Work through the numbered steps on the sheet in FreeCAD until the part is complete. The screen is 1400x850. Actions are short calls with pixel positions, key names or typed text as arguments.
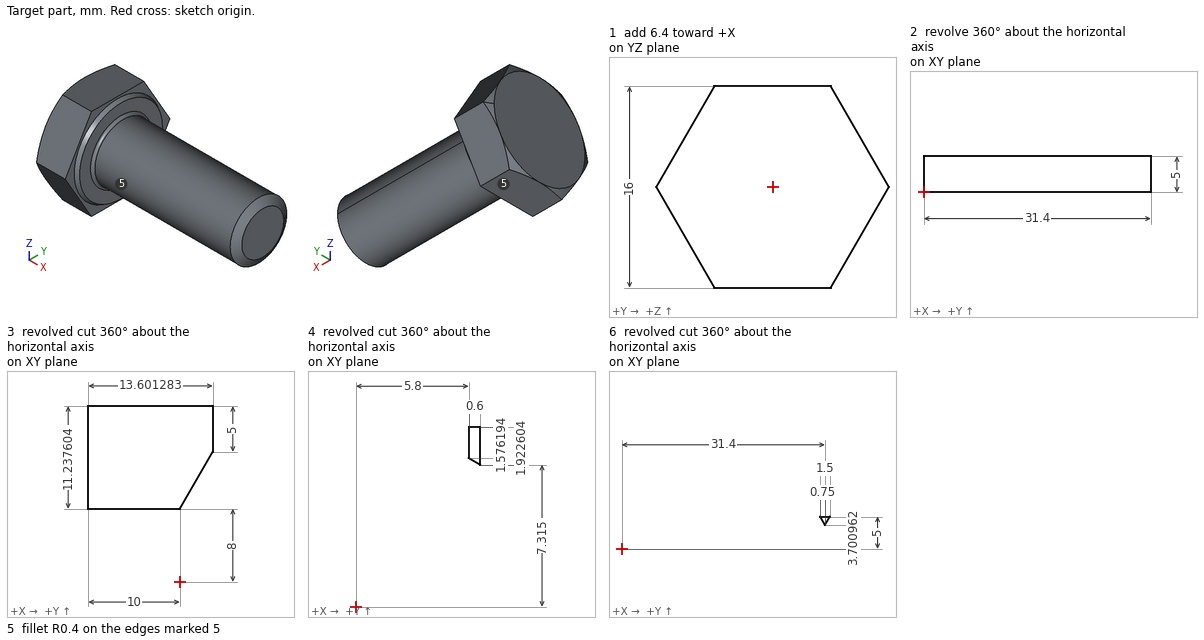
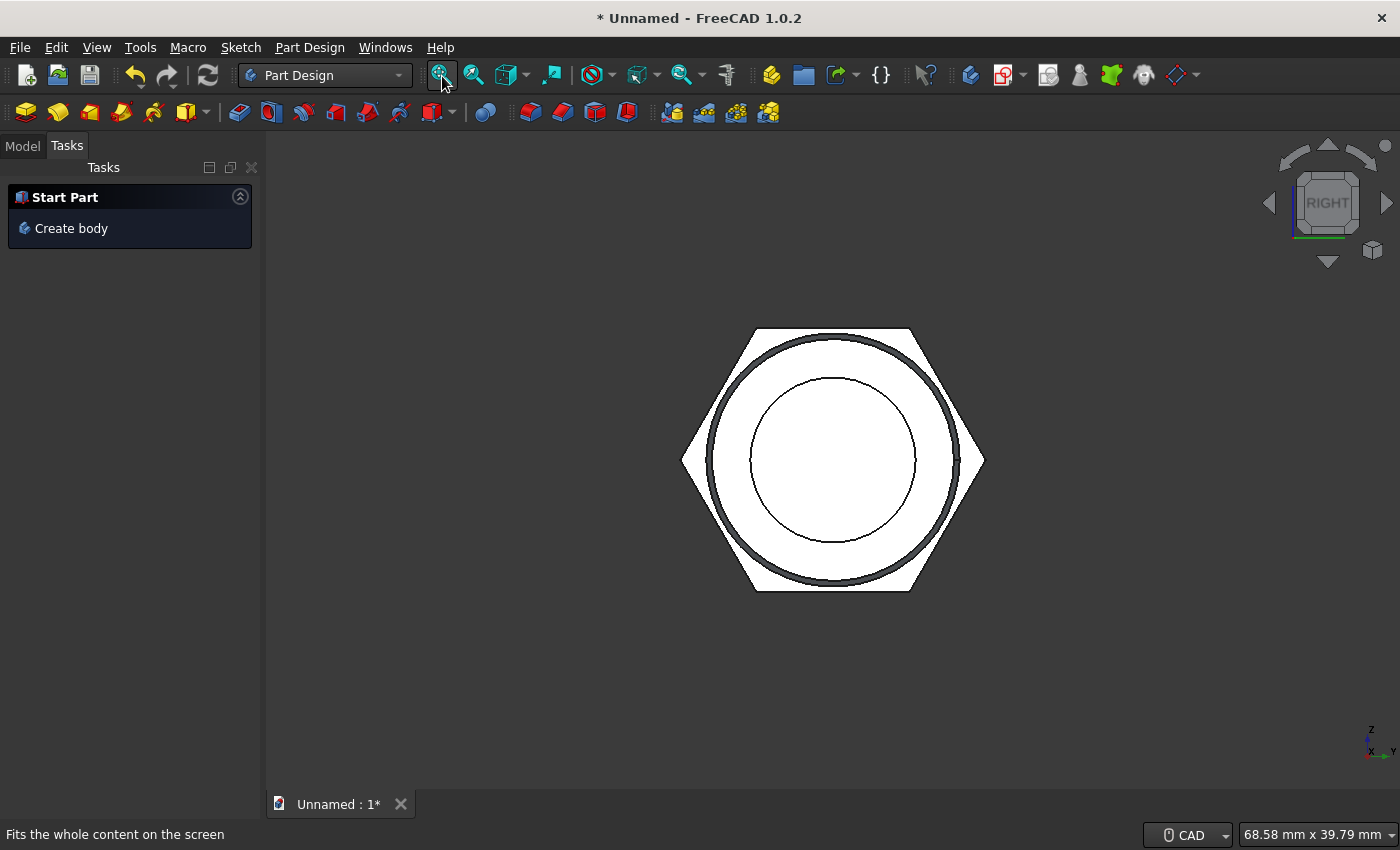
key(5)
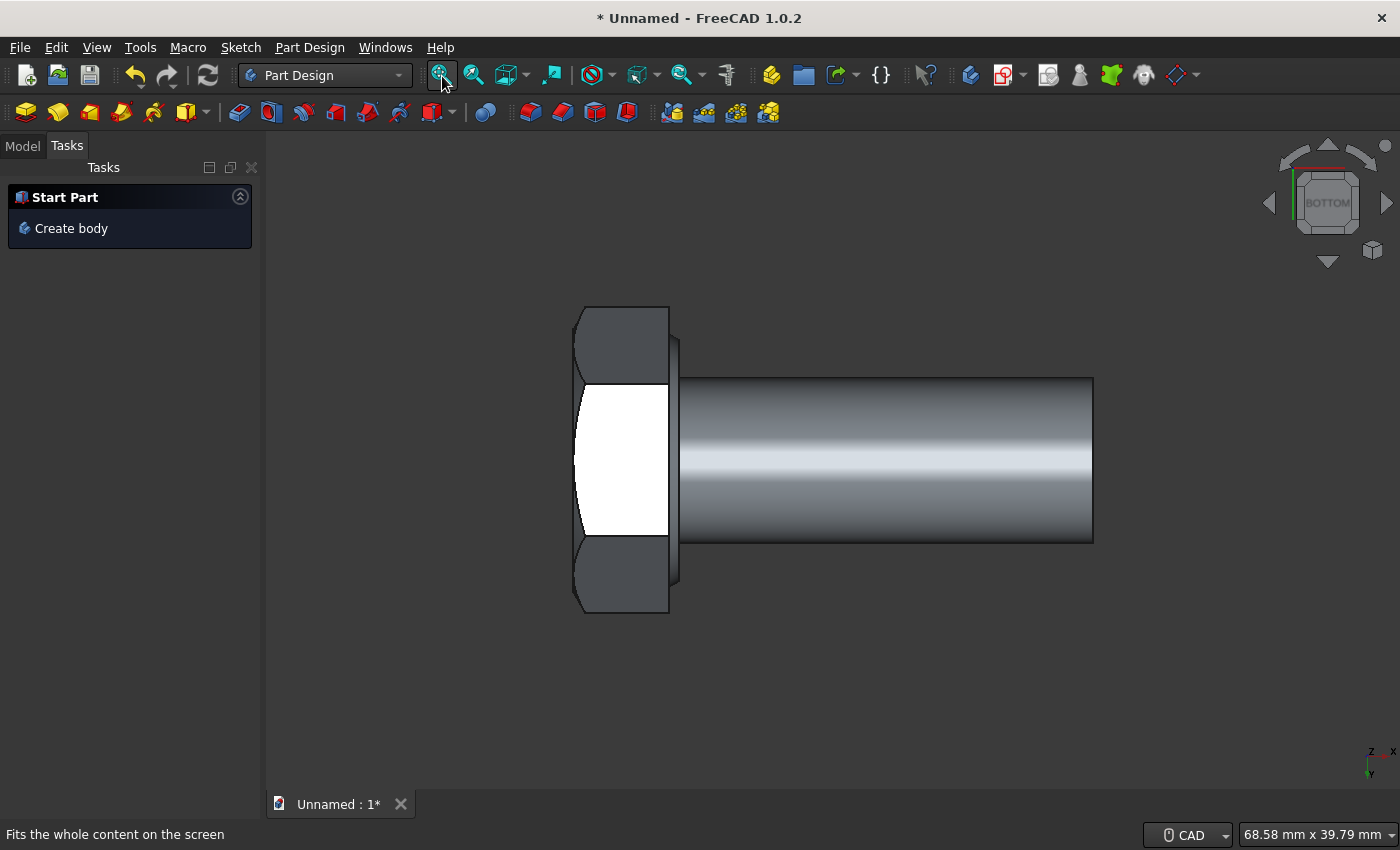
key(4)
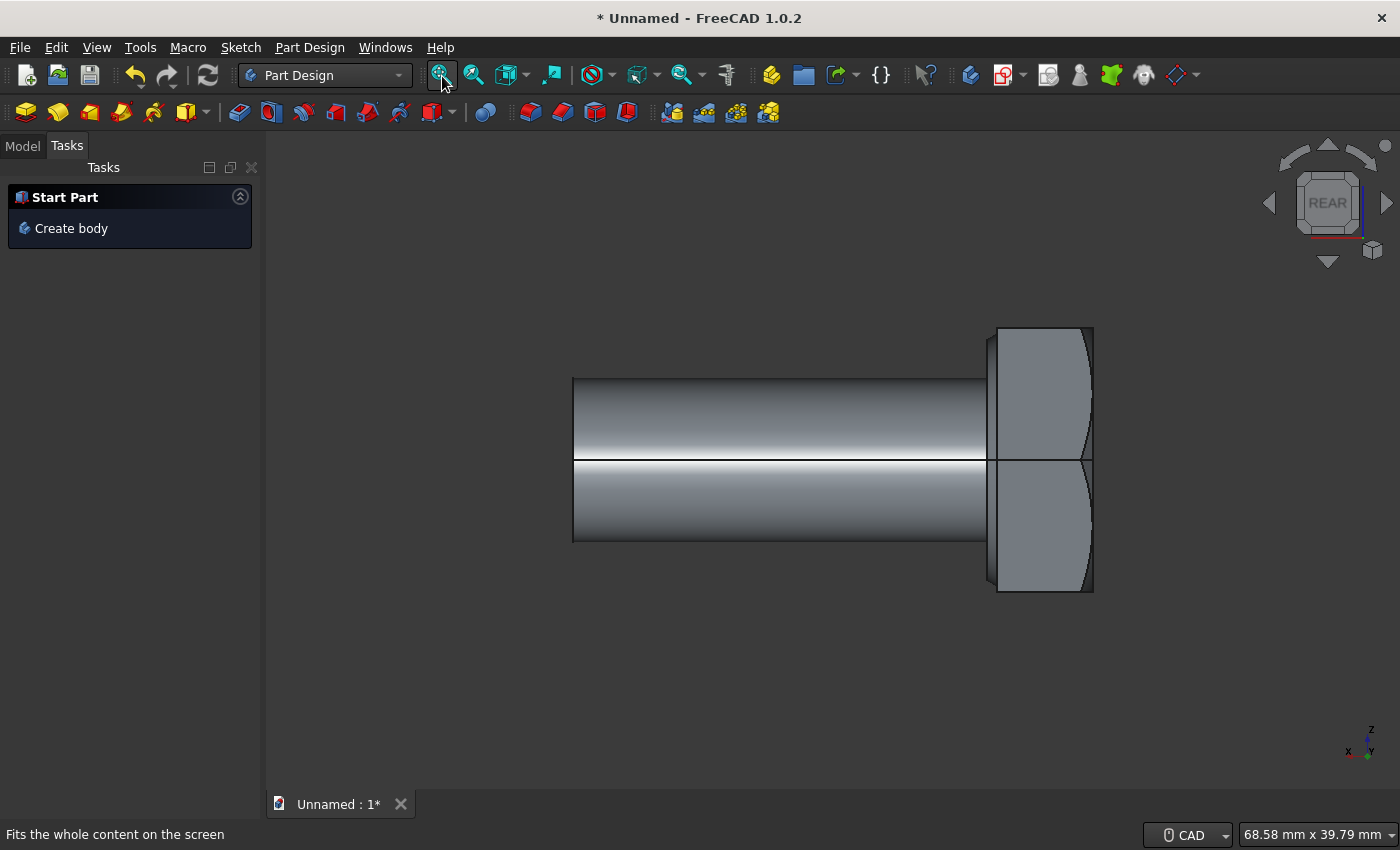
key(6)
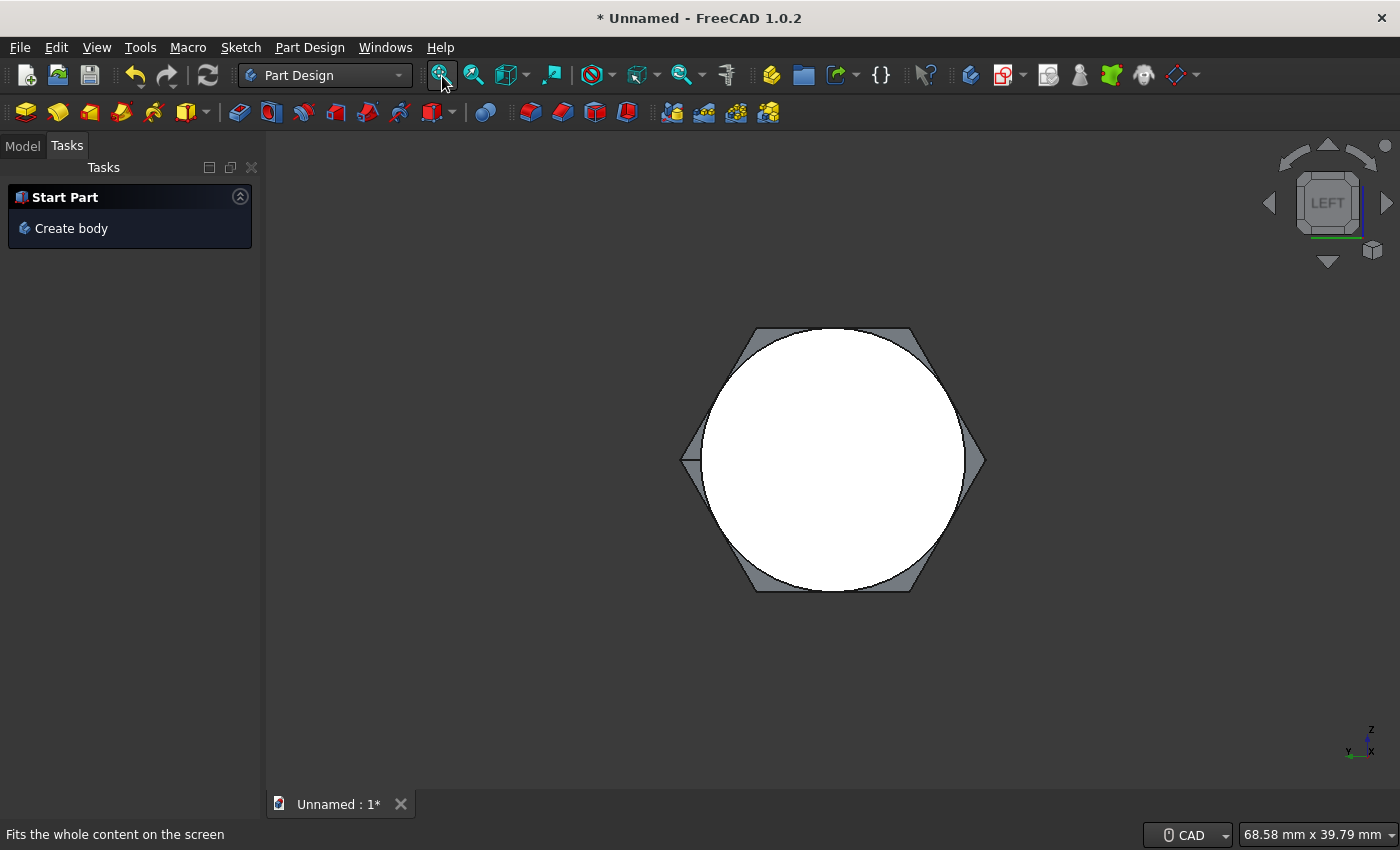
click(442, 76)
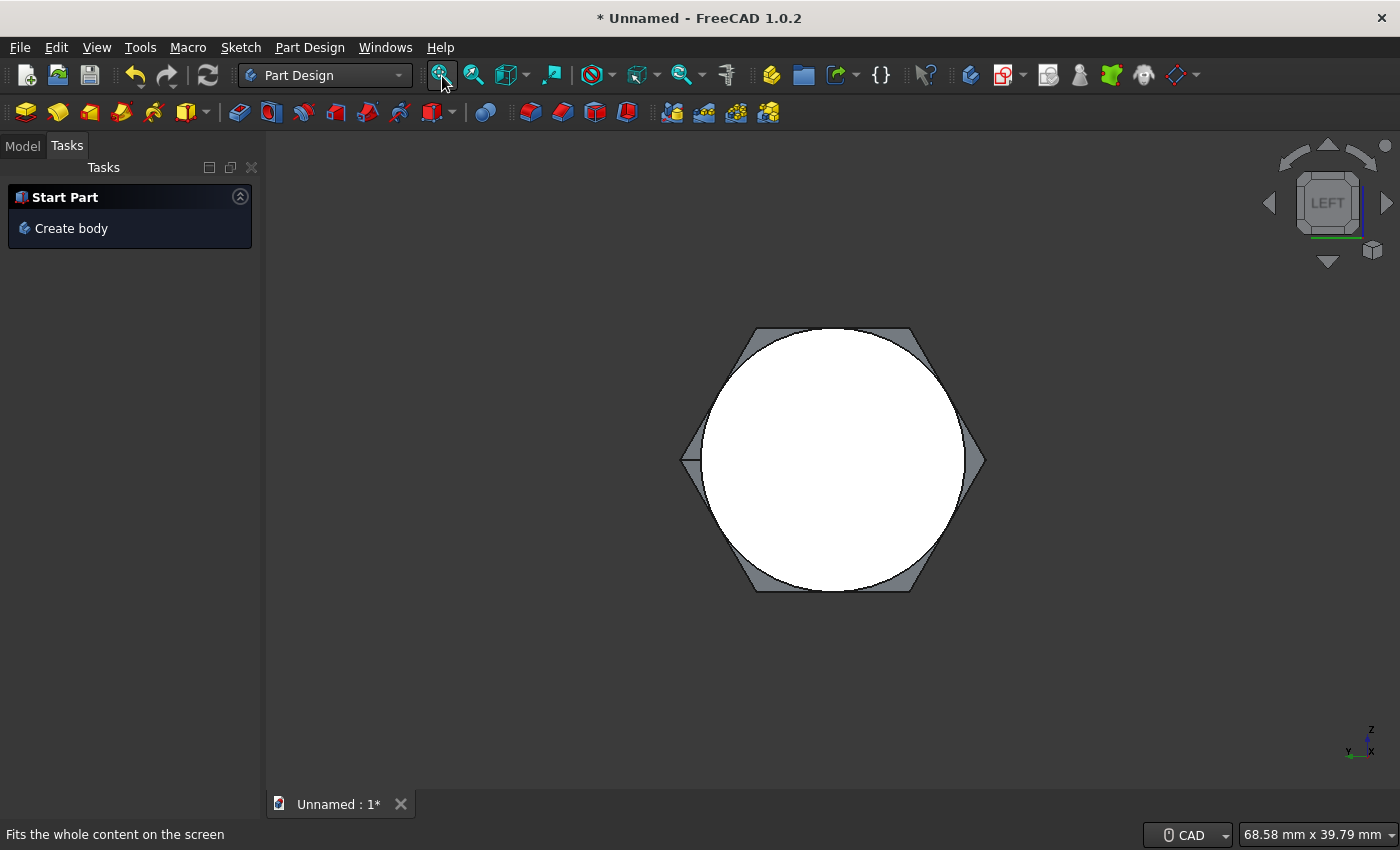
key(v)
key(3)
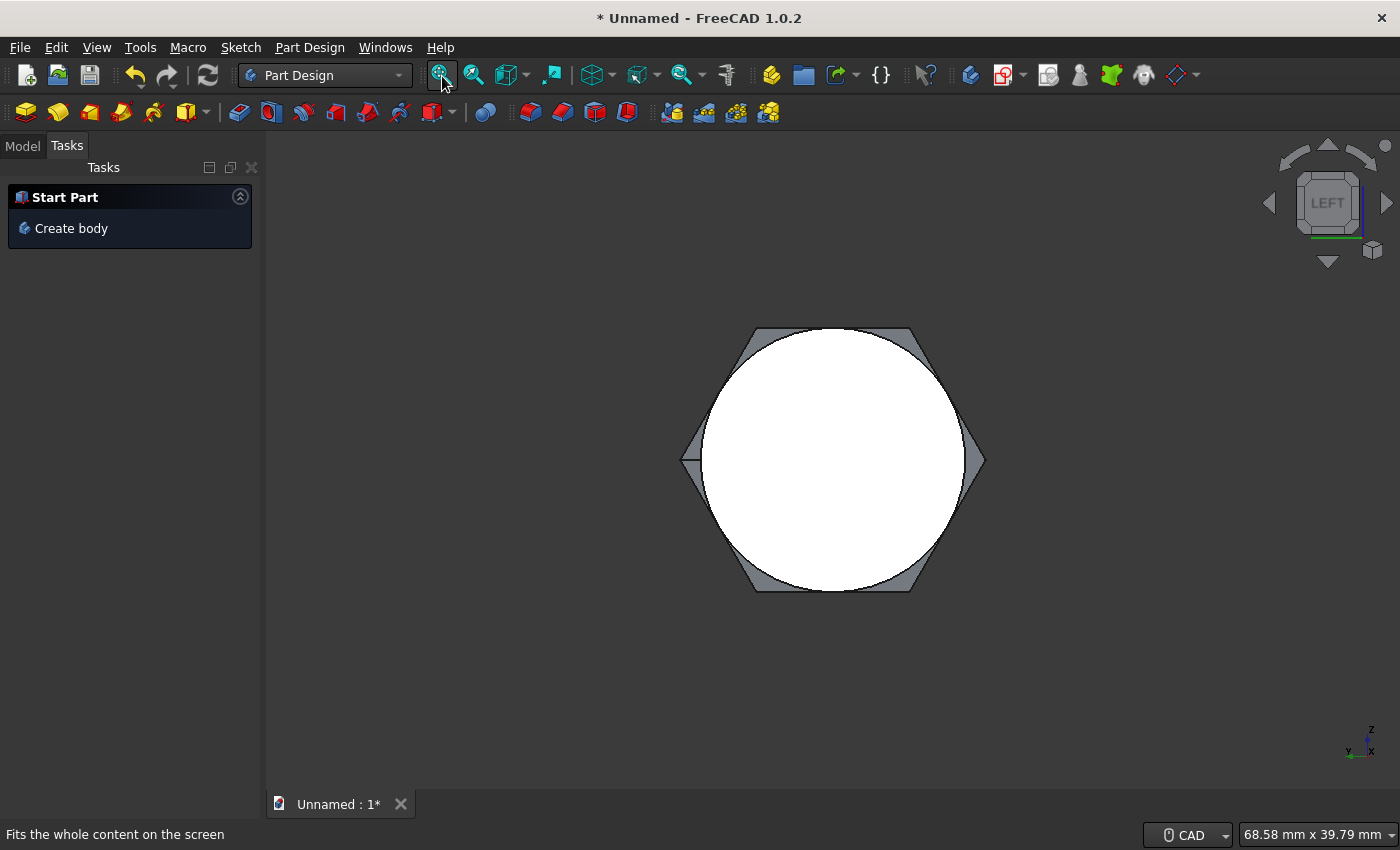
key(0)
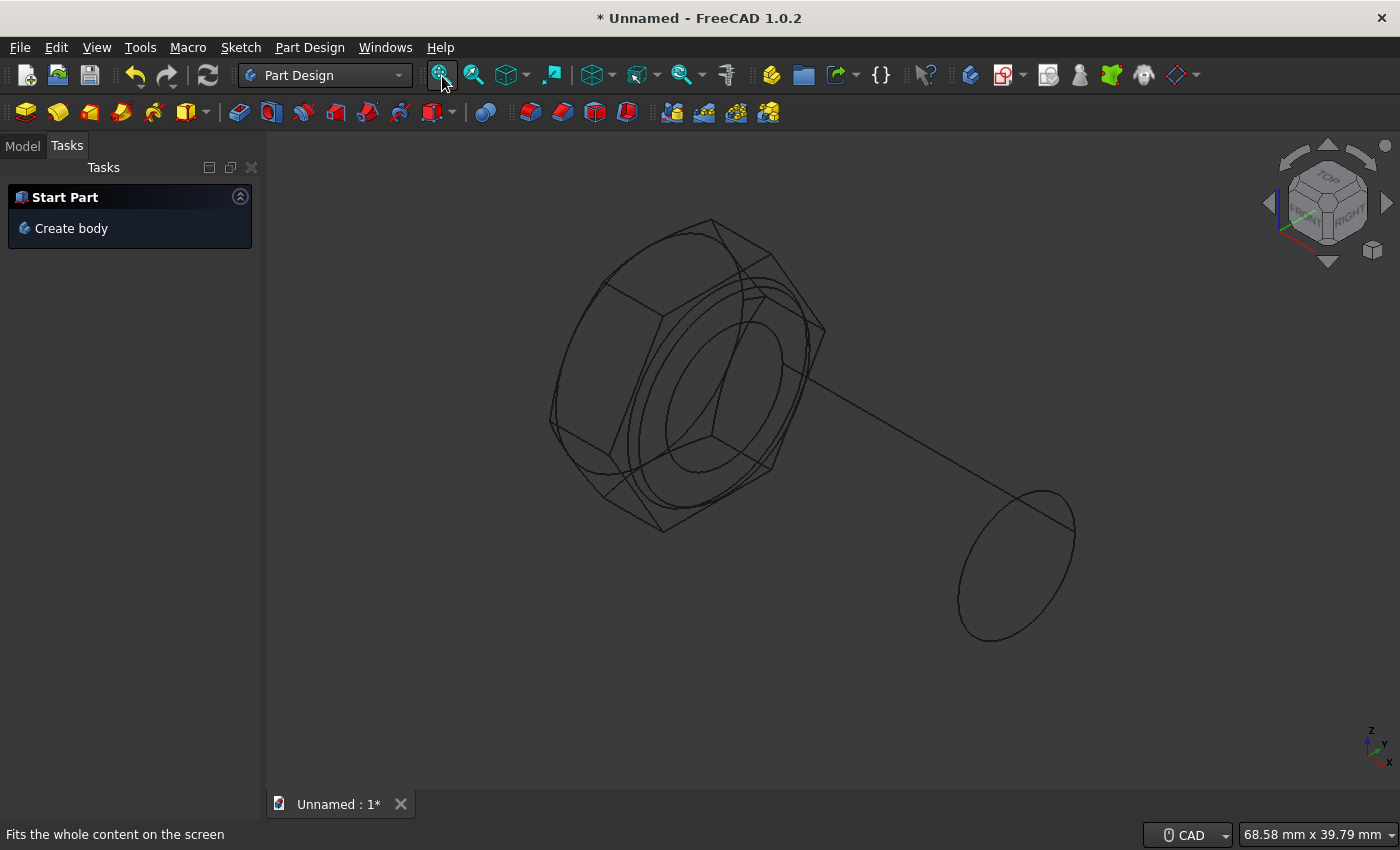
click(666, 430)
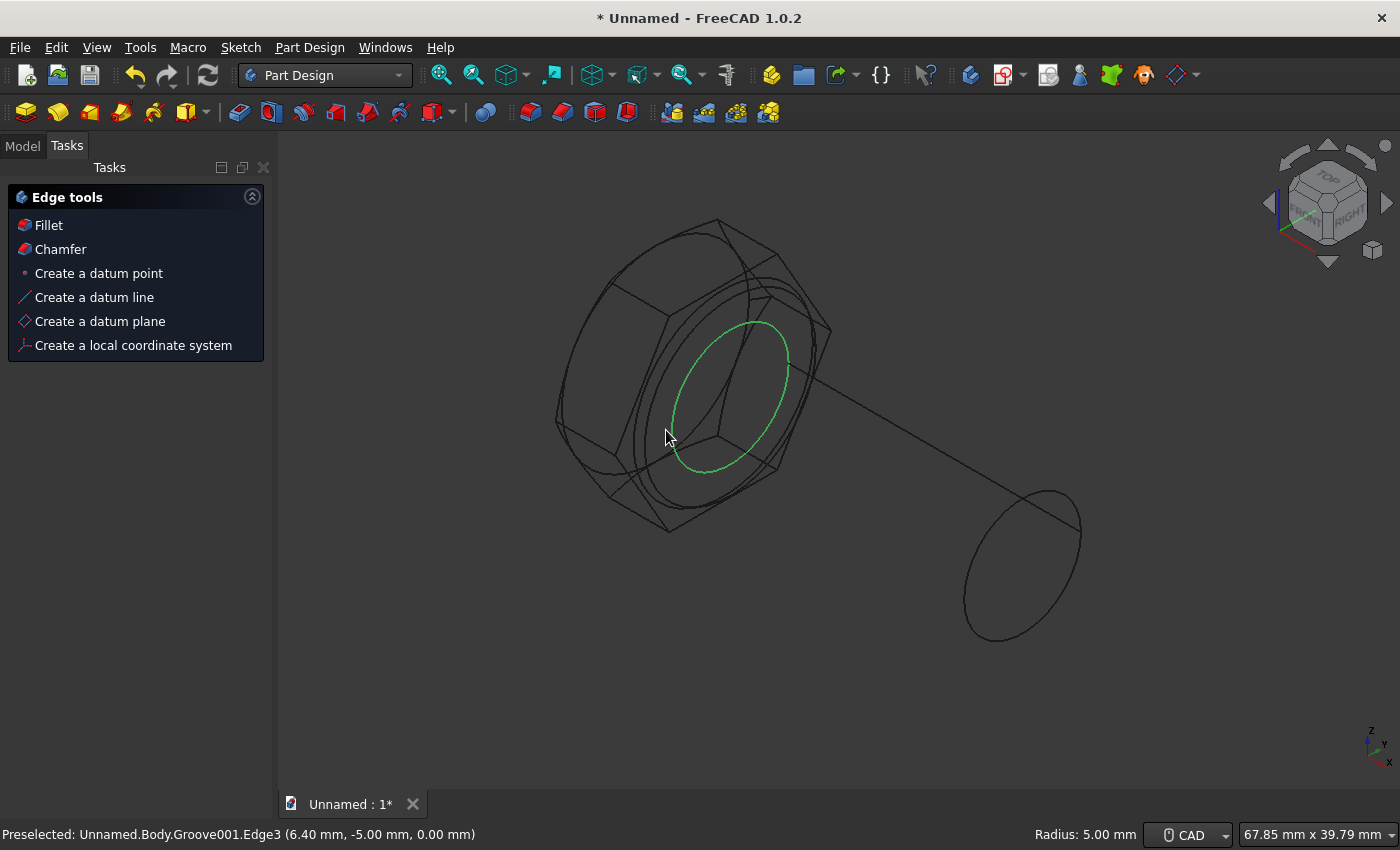
key(v)
key(1)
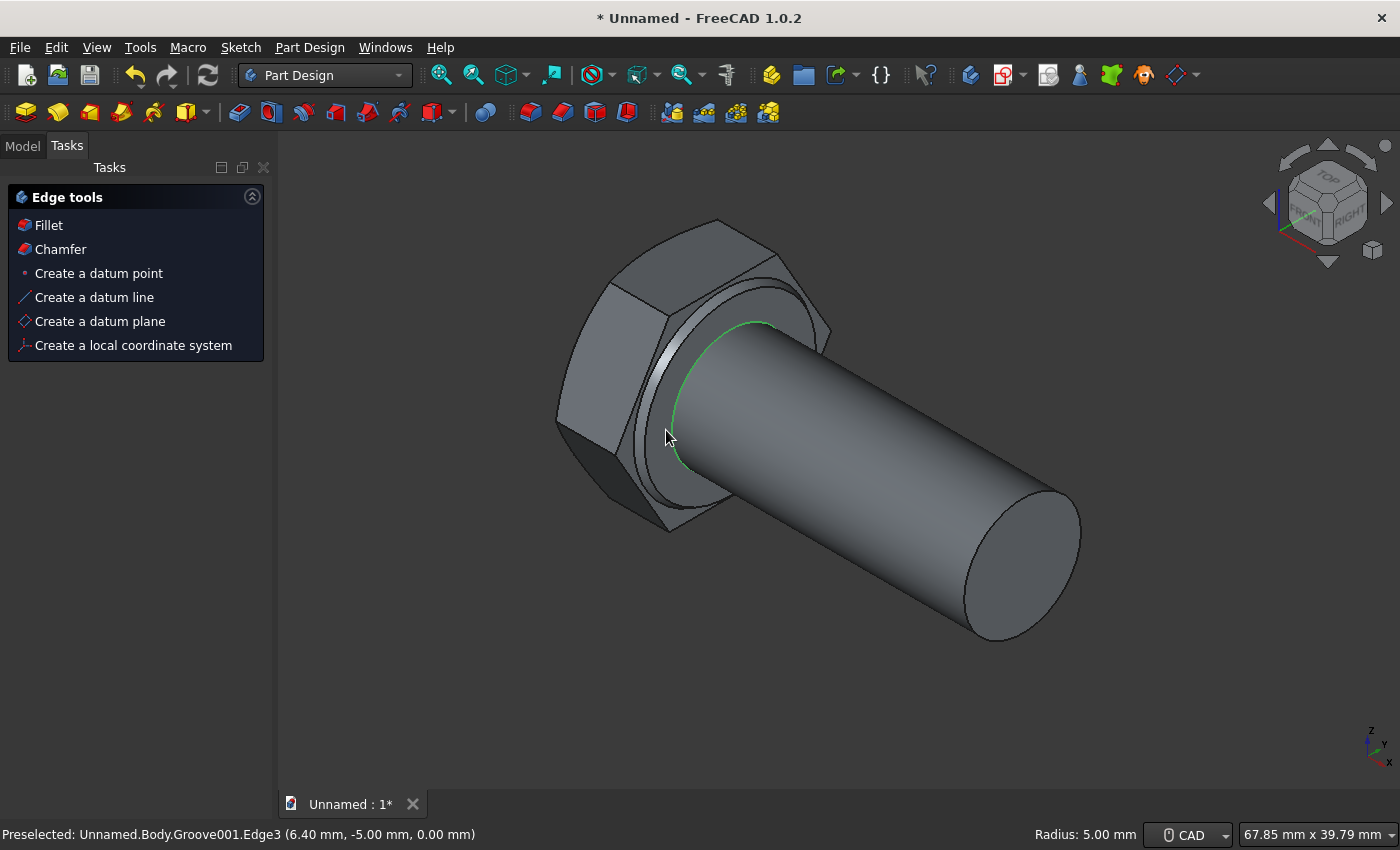
click(532, 112)